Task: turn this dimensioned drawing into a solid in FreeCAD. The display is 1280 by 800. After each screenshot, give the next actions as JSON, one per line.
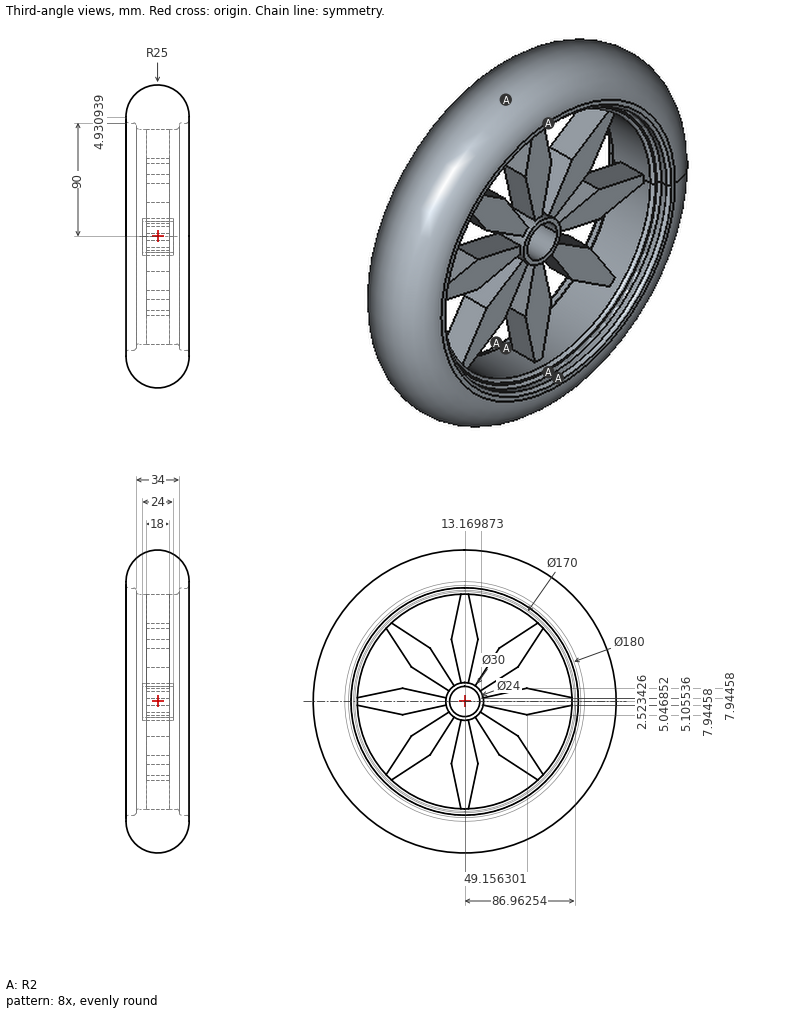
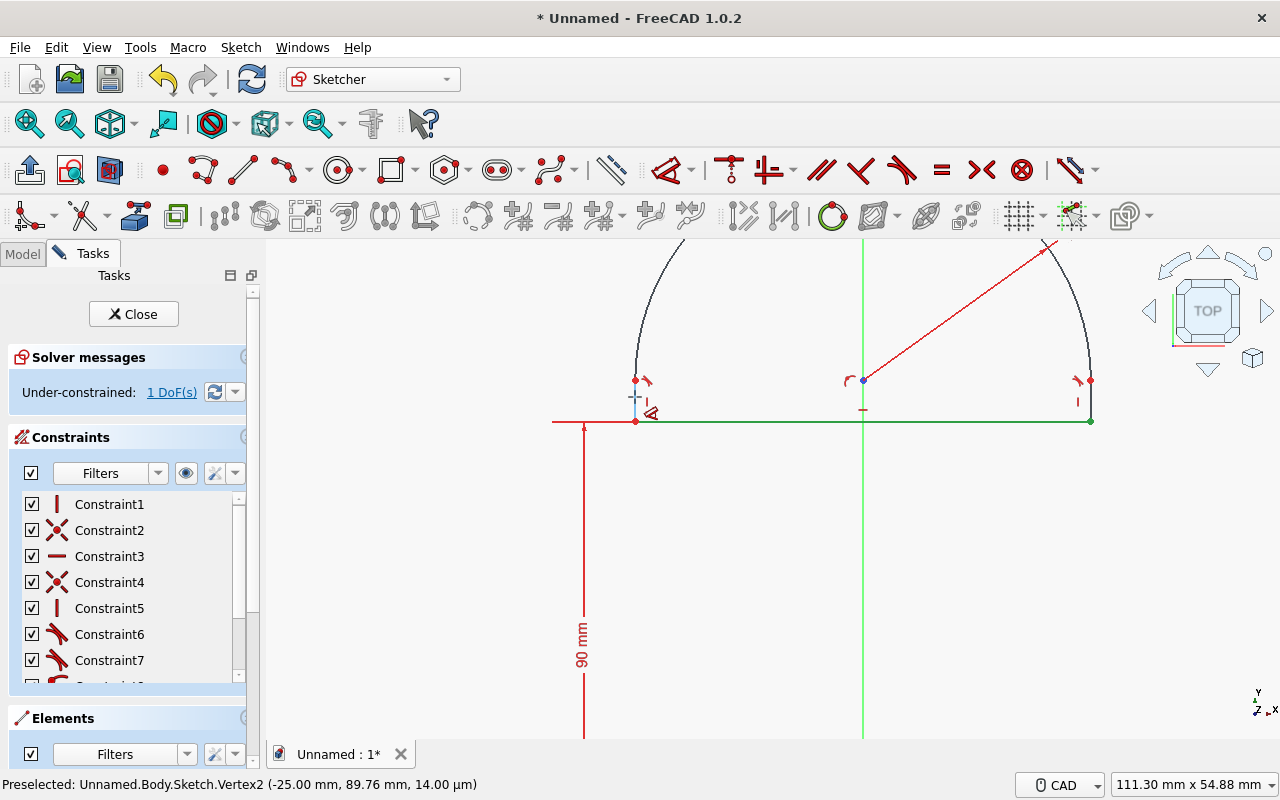
{"action": "left_click", "coordinate": [635, 397]}
{"action": "left_click", "coordinate": [601, 401]}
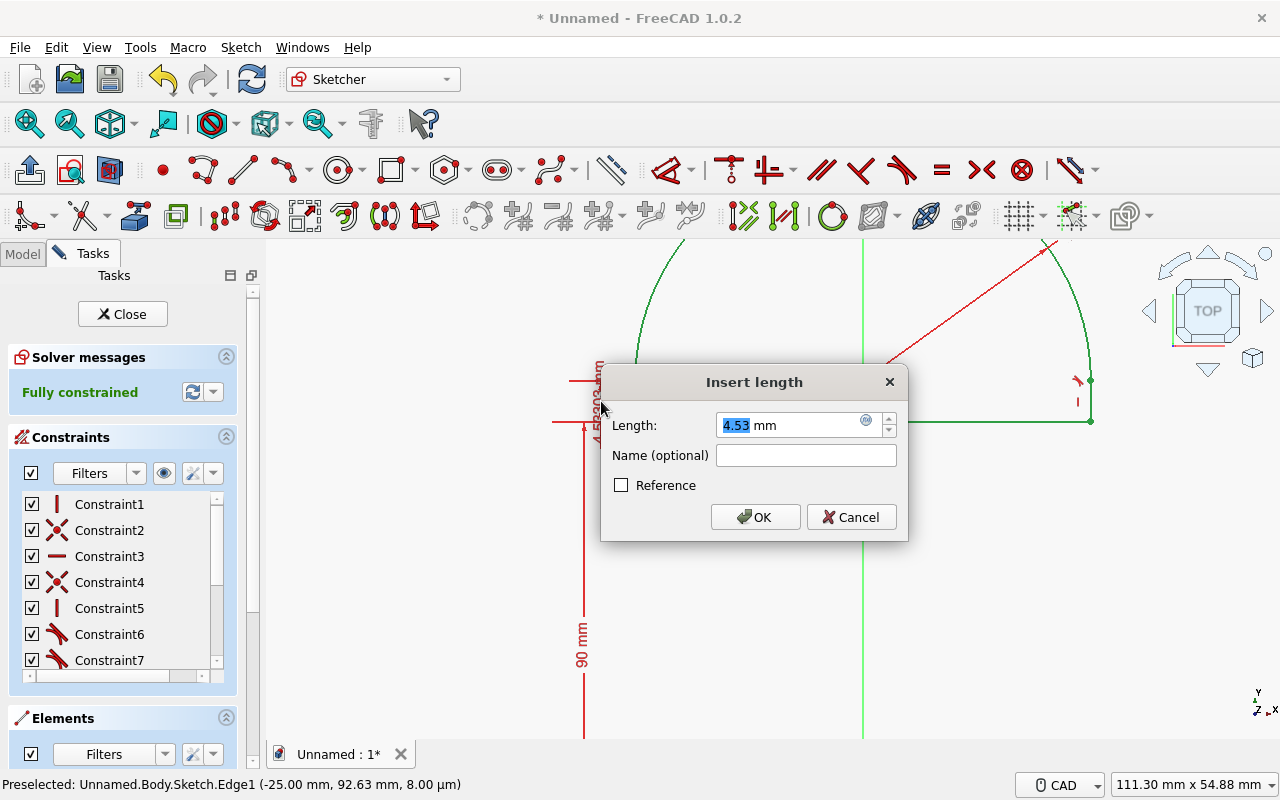
{"action": "type", "text": "4.930939"}
{"action": "key", "text": "Return"}
{"action": "key", "text": "Escape"}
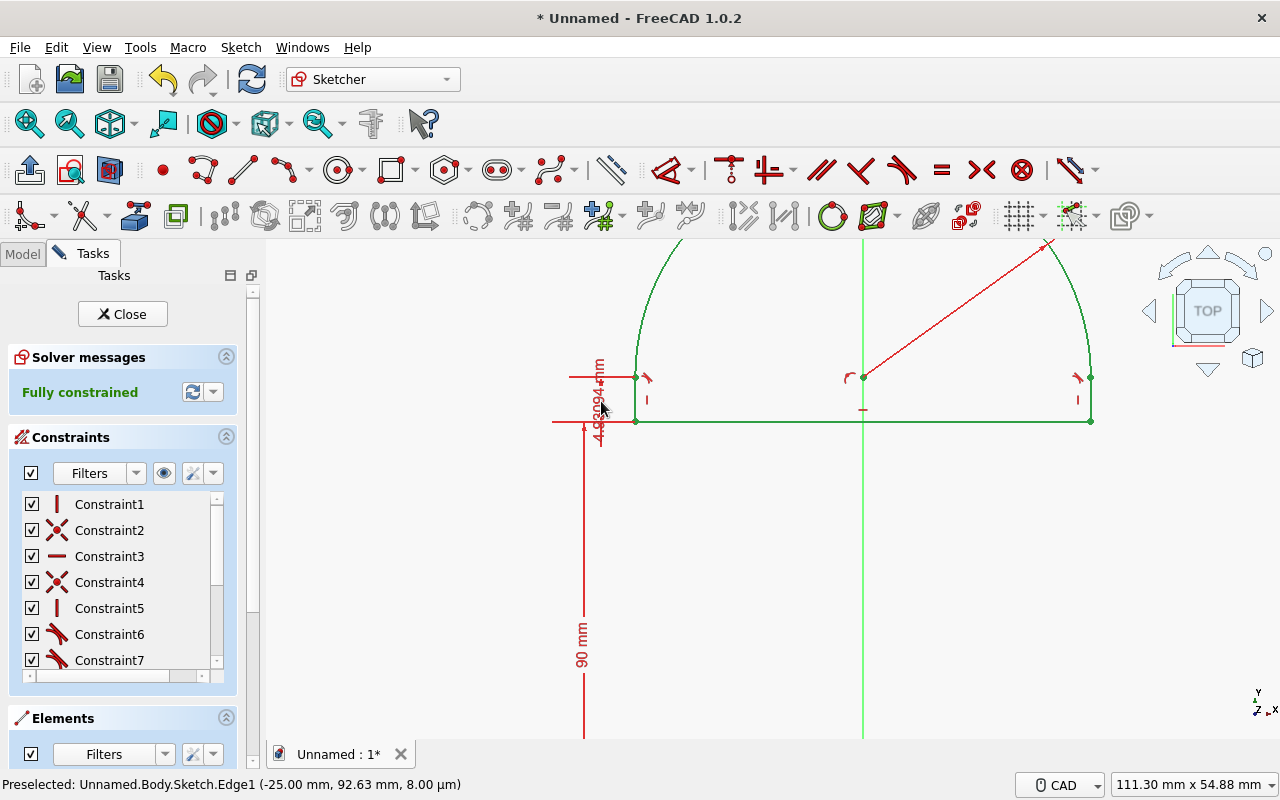
{"action": "left_click", "coordinate": [123, 314]}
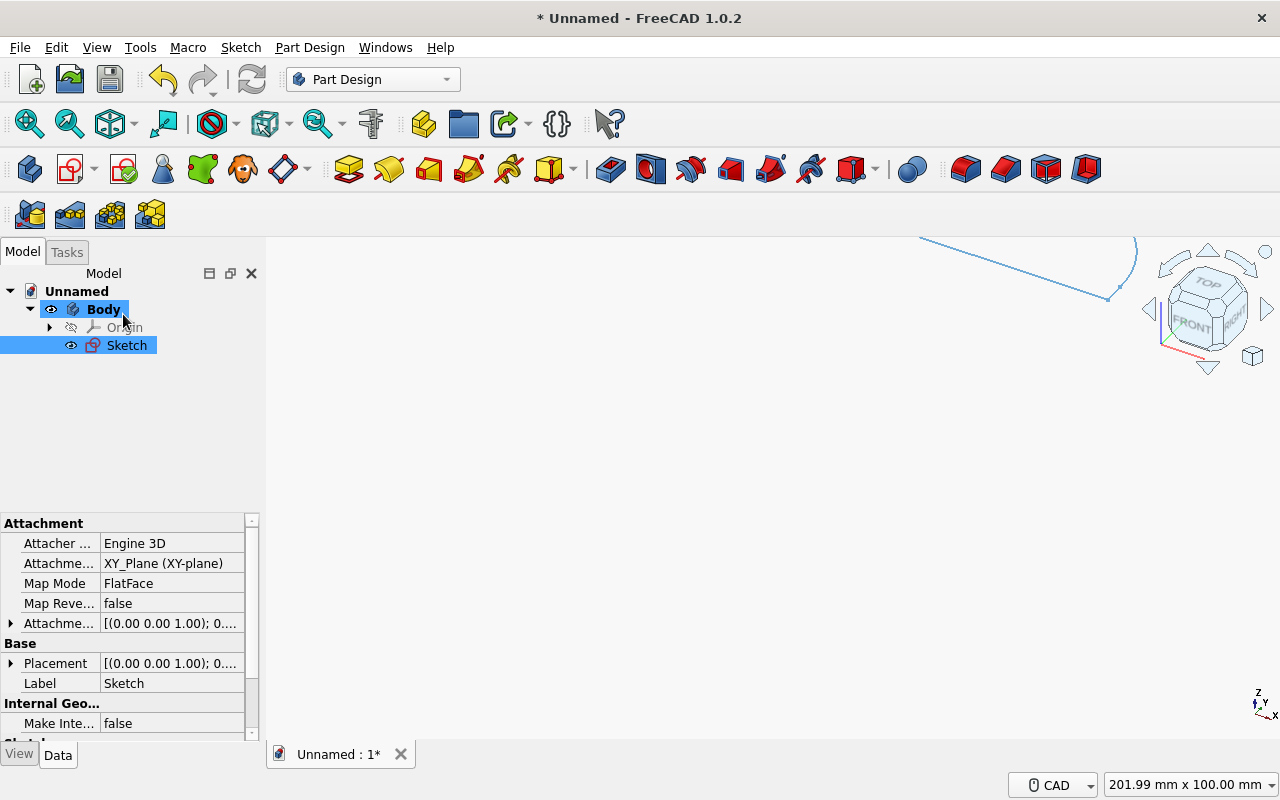
{"action": "left_click", "coordinate": [390, 170]}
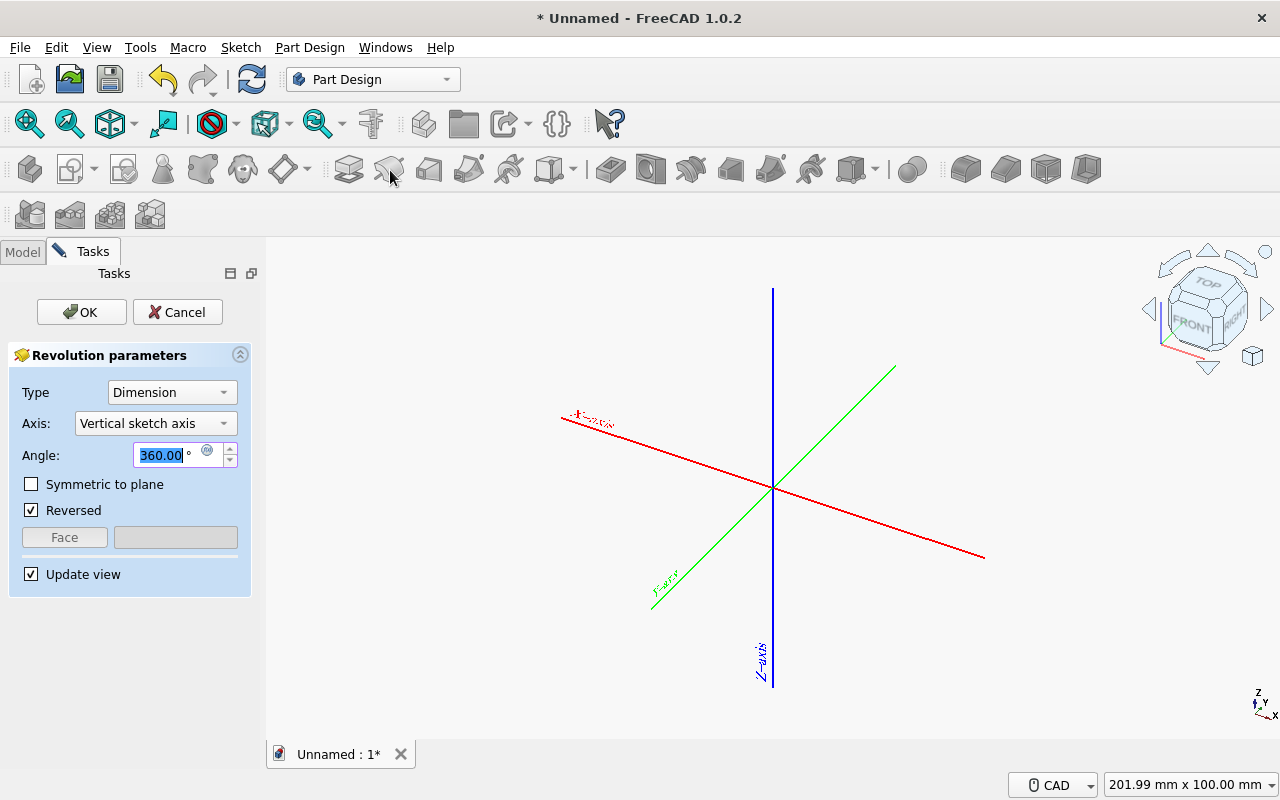
{"action": "left_click", "coordinate": [156, 424]}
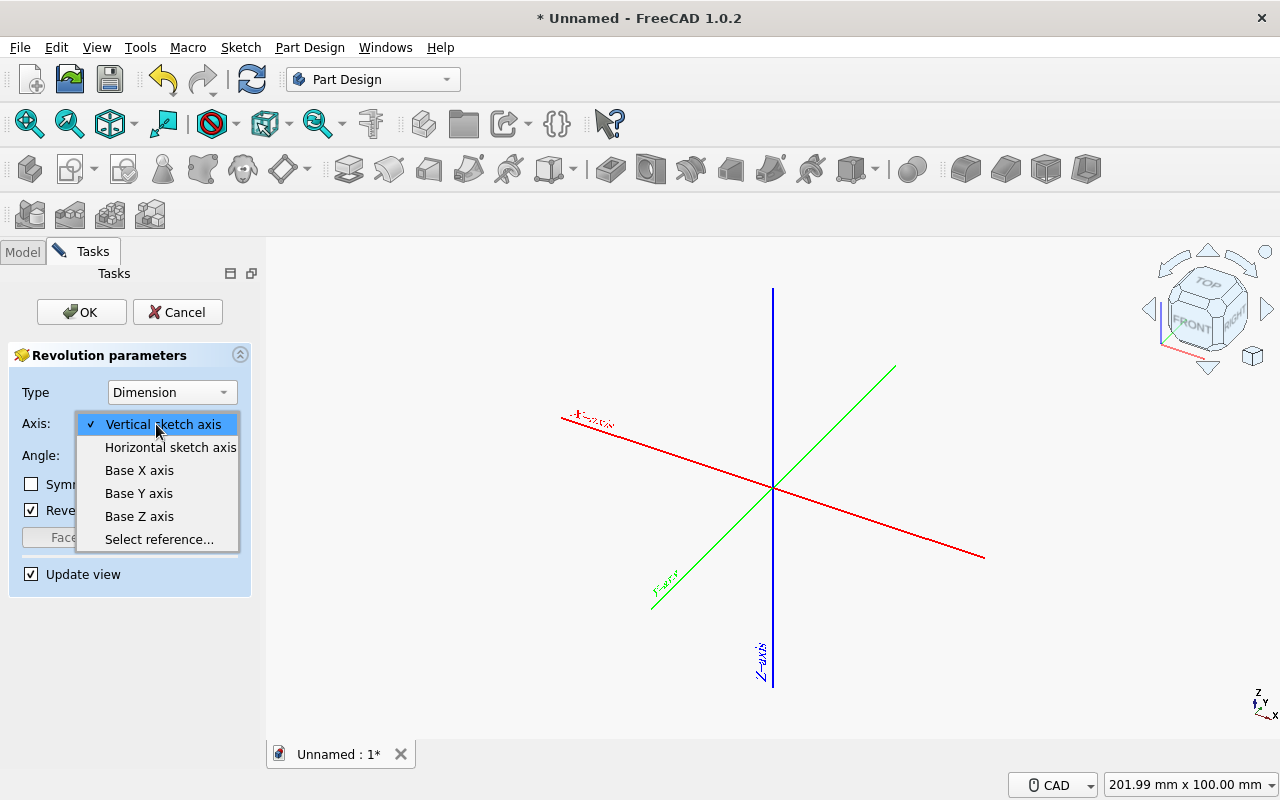
{"action": "left_click", "coordinate": [156, 448]}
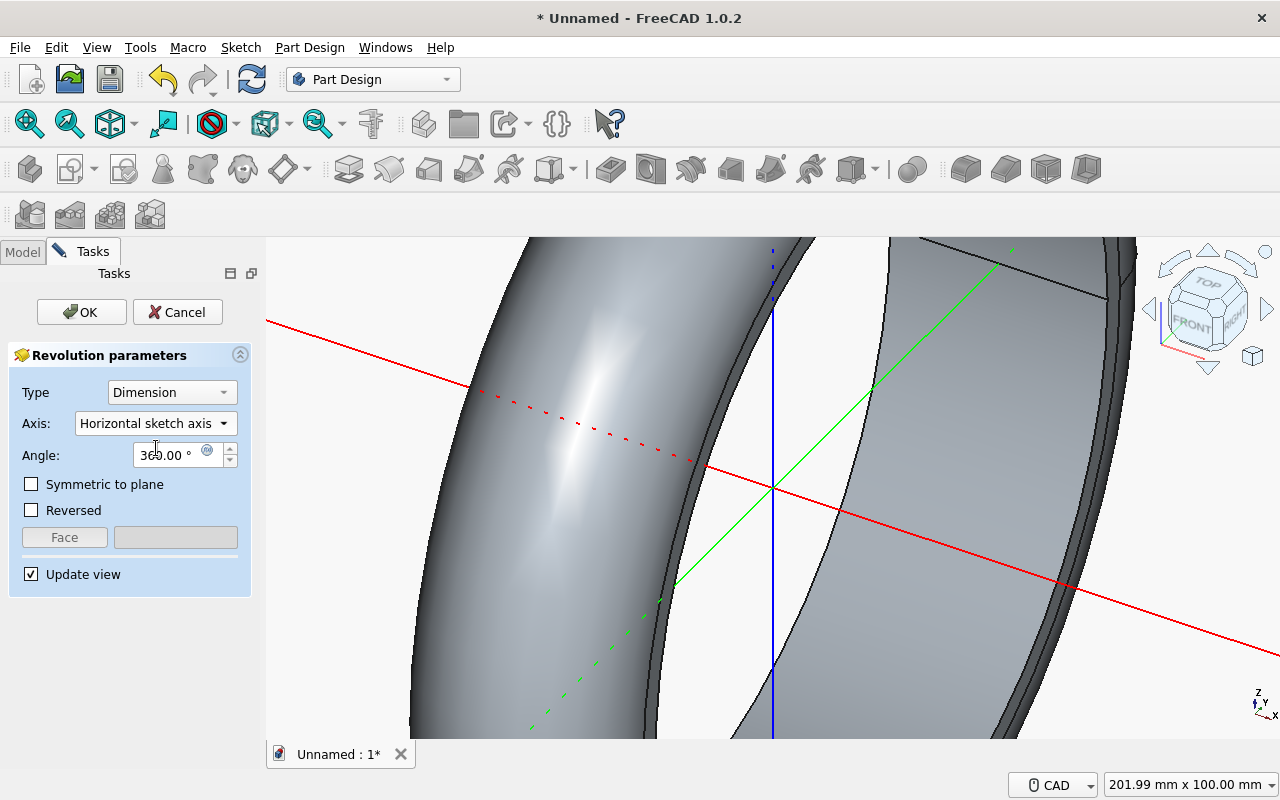
{"action": "left_click", "coordinate": [82, 312]}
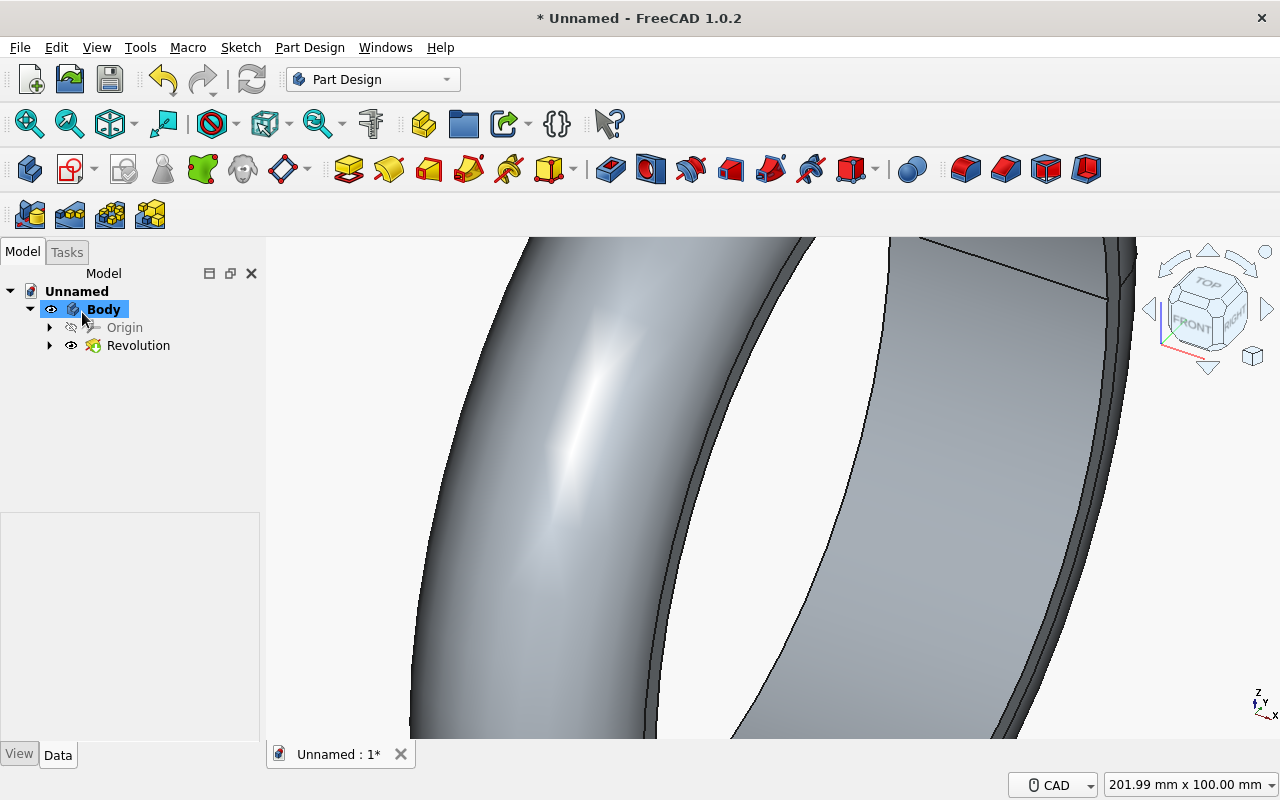
{"action": "key", "text": "v f"}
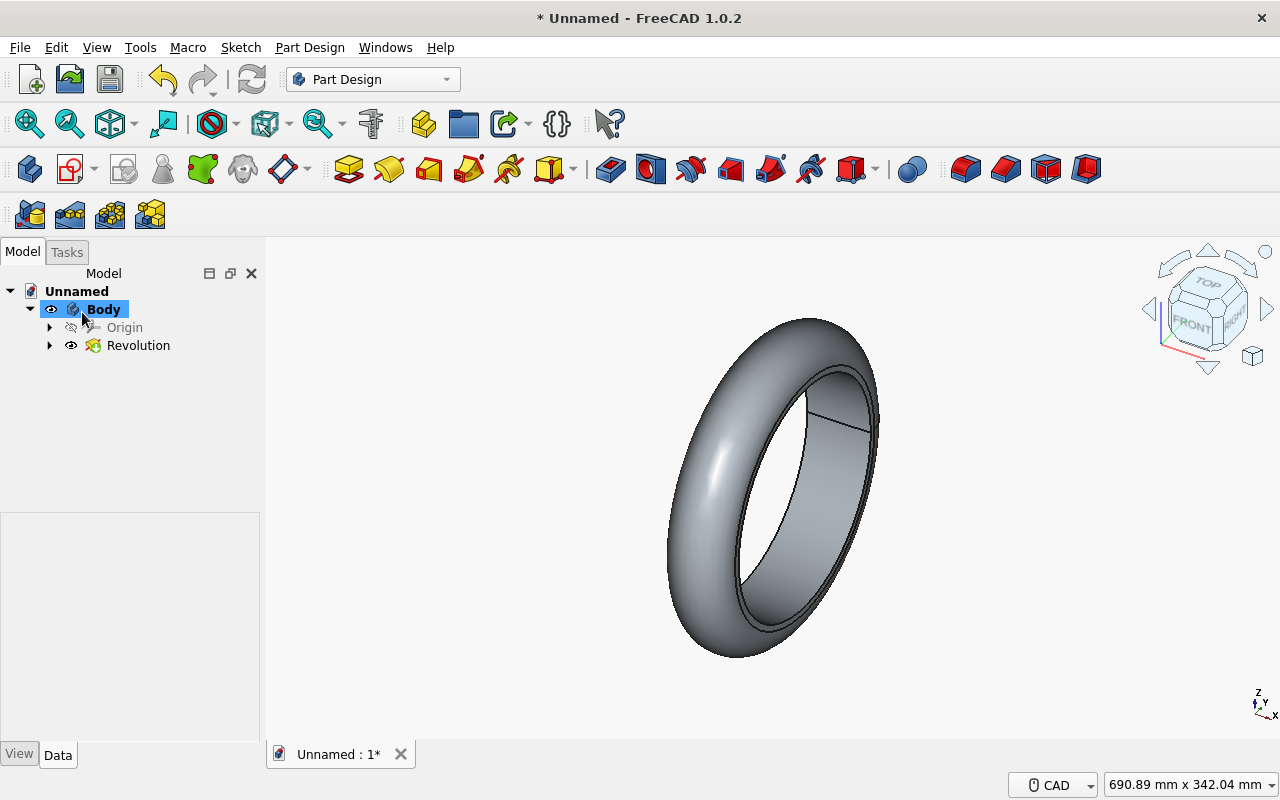
{"action": "left_click", "coordinate": [70, 170]}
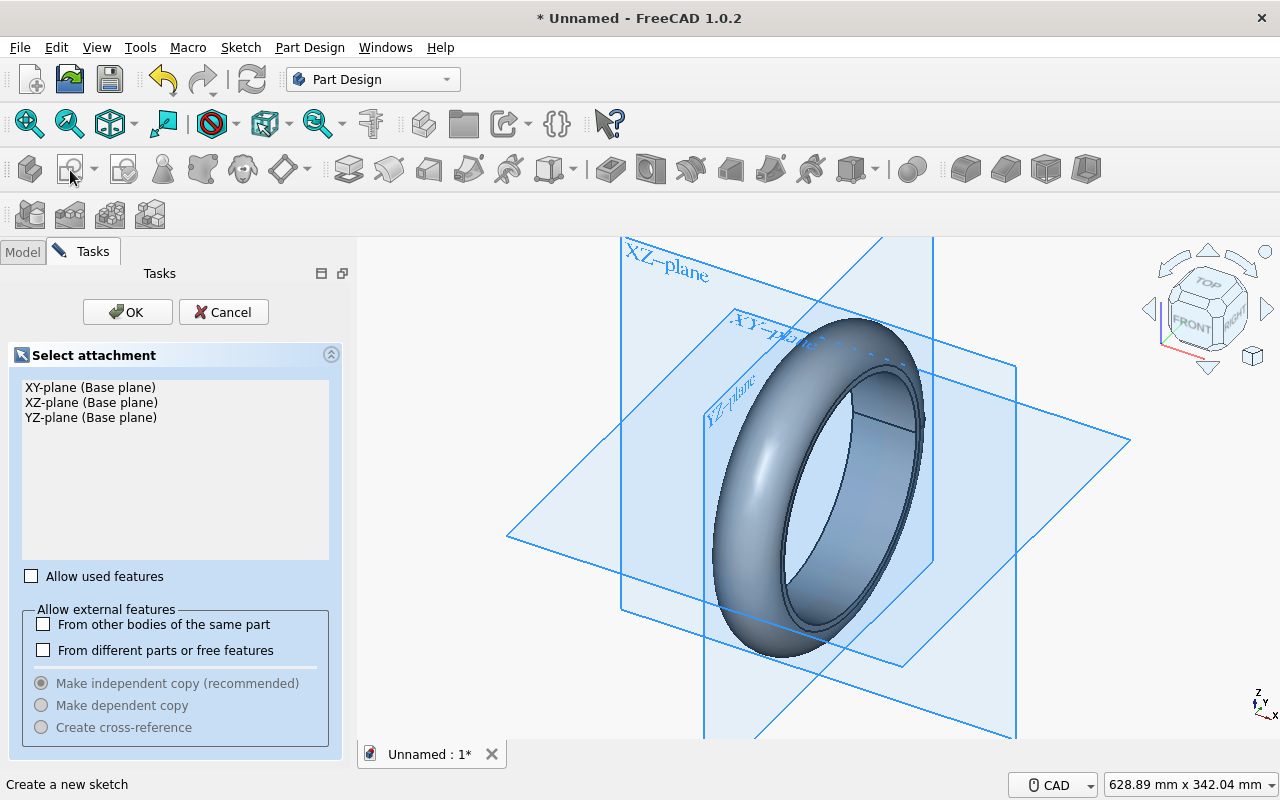
{"action": "left_click", "coordinate": [82, 418]}